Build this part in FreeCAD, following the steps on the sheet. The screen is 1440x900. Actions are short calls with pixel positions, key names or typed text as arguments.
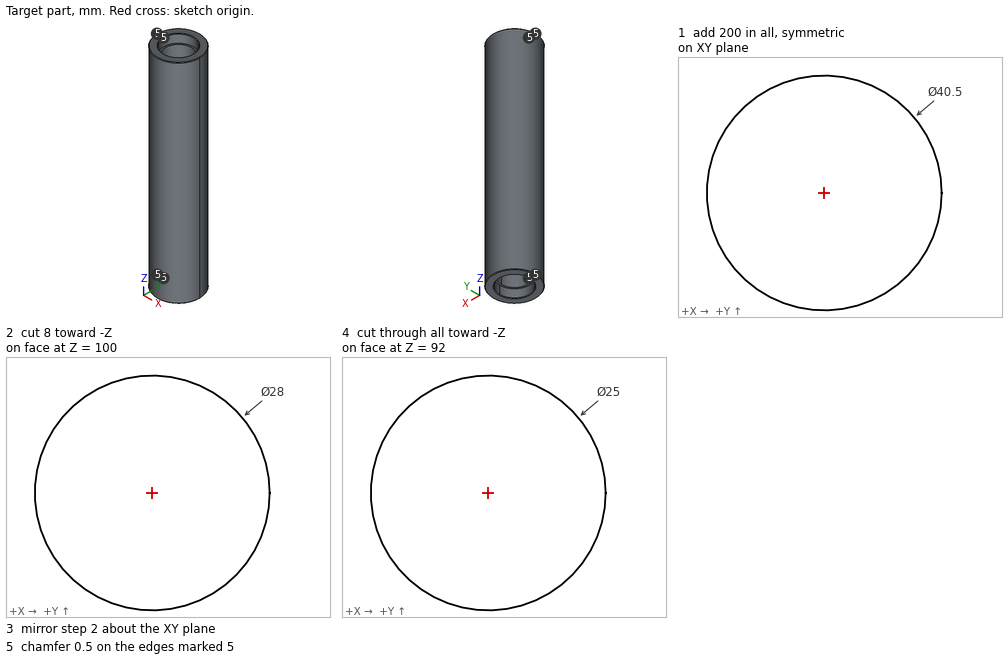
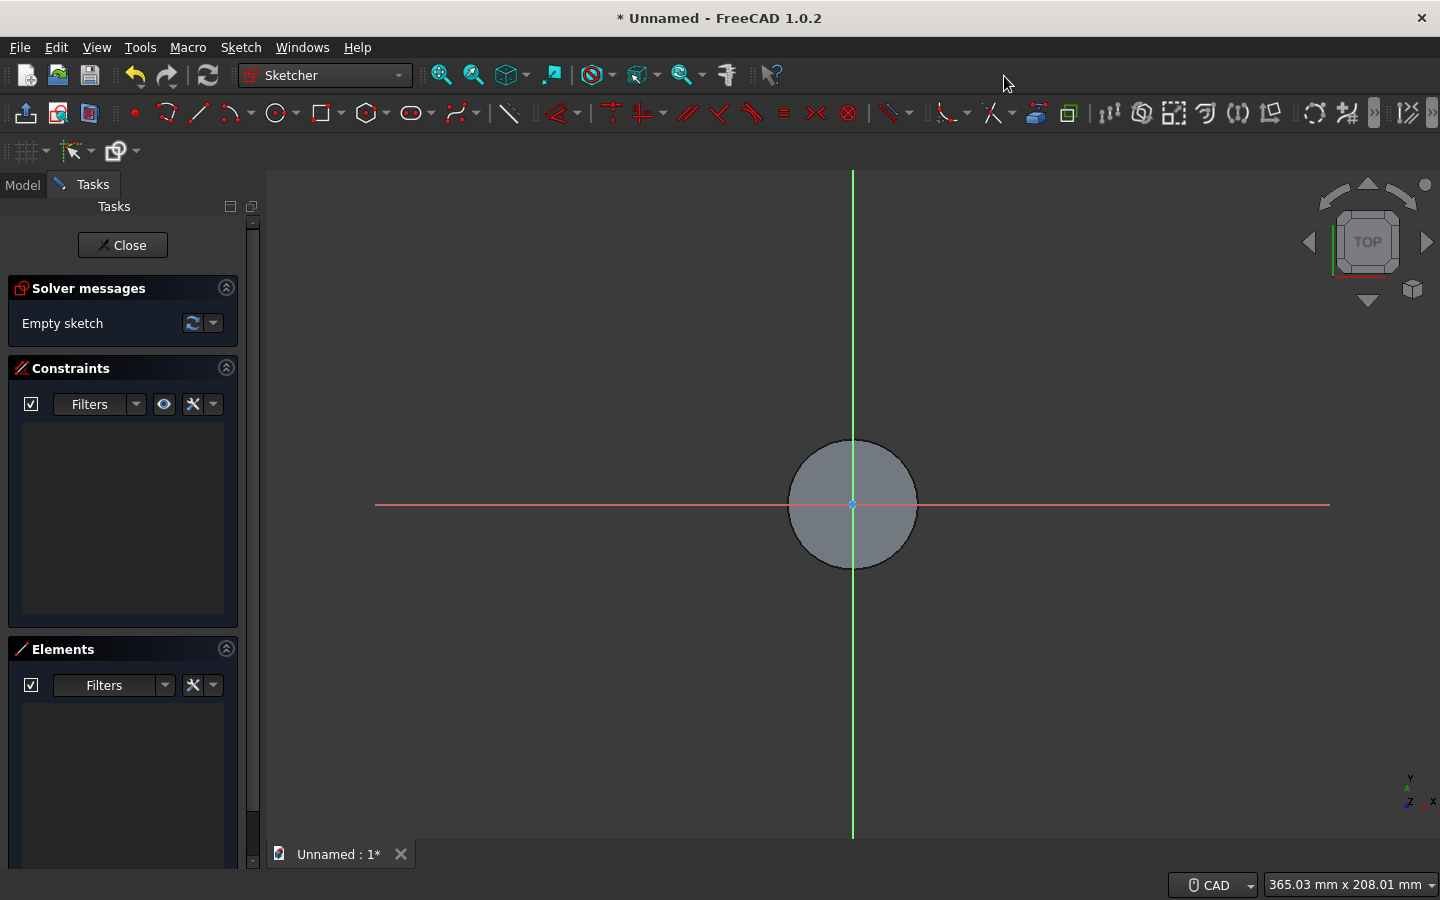
scroll(870, 504, up, 8)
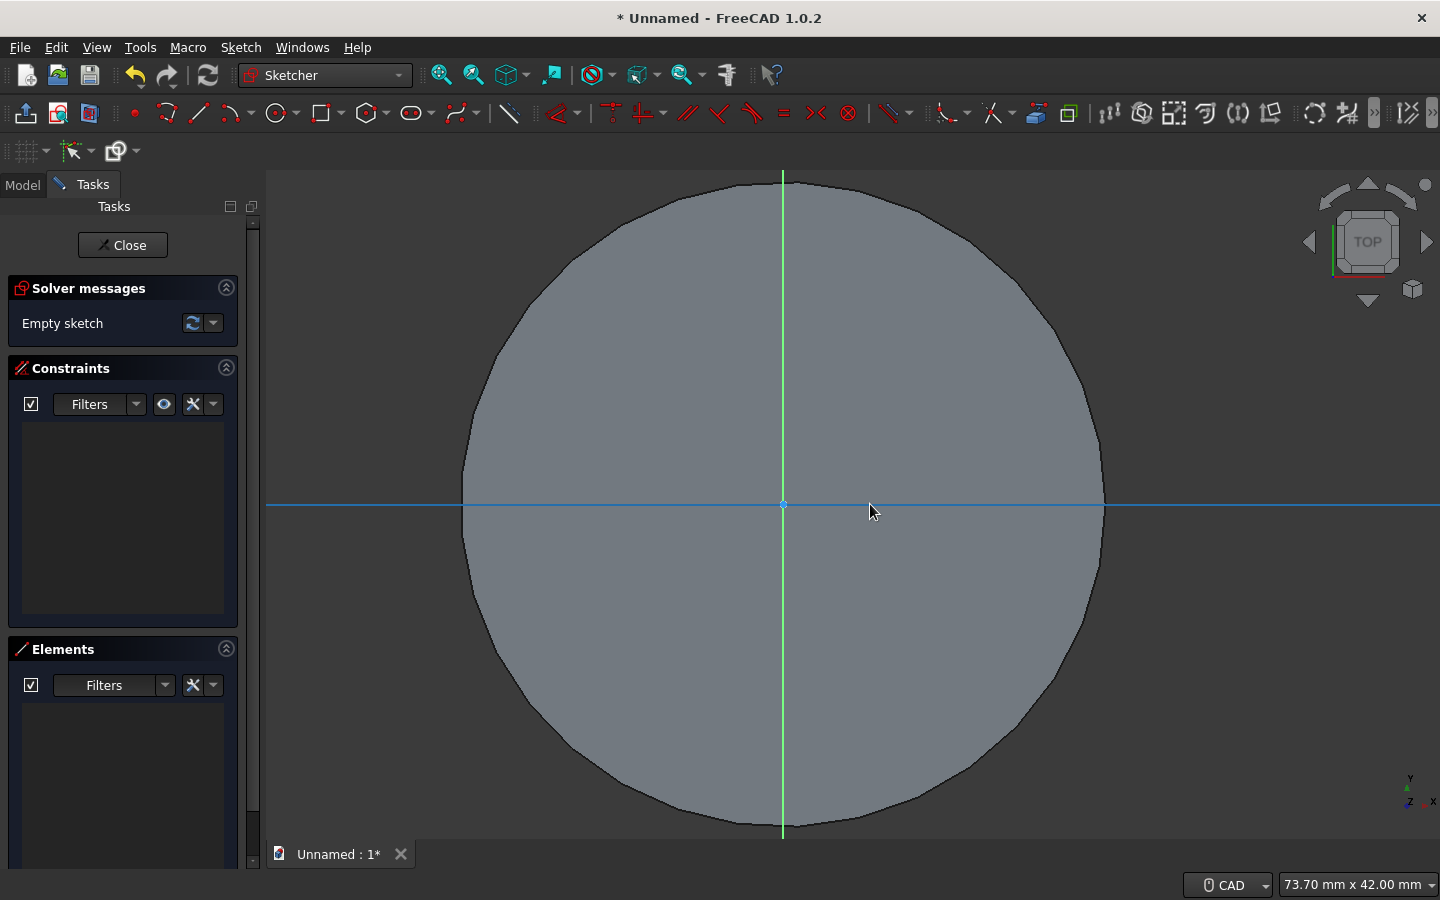
click(276, 114)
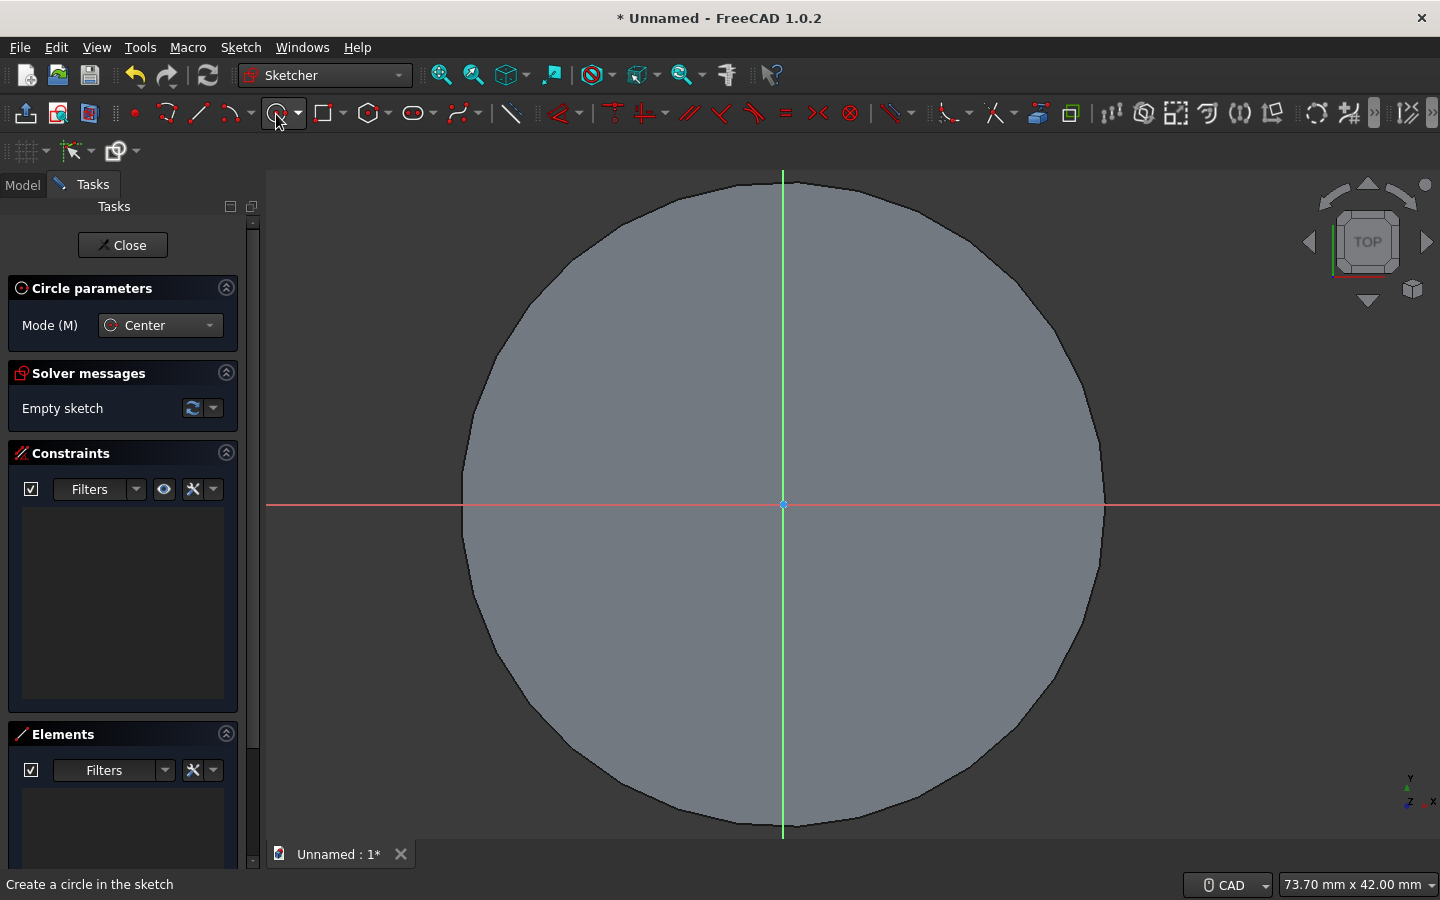
click(783, 504)
move(941, 347)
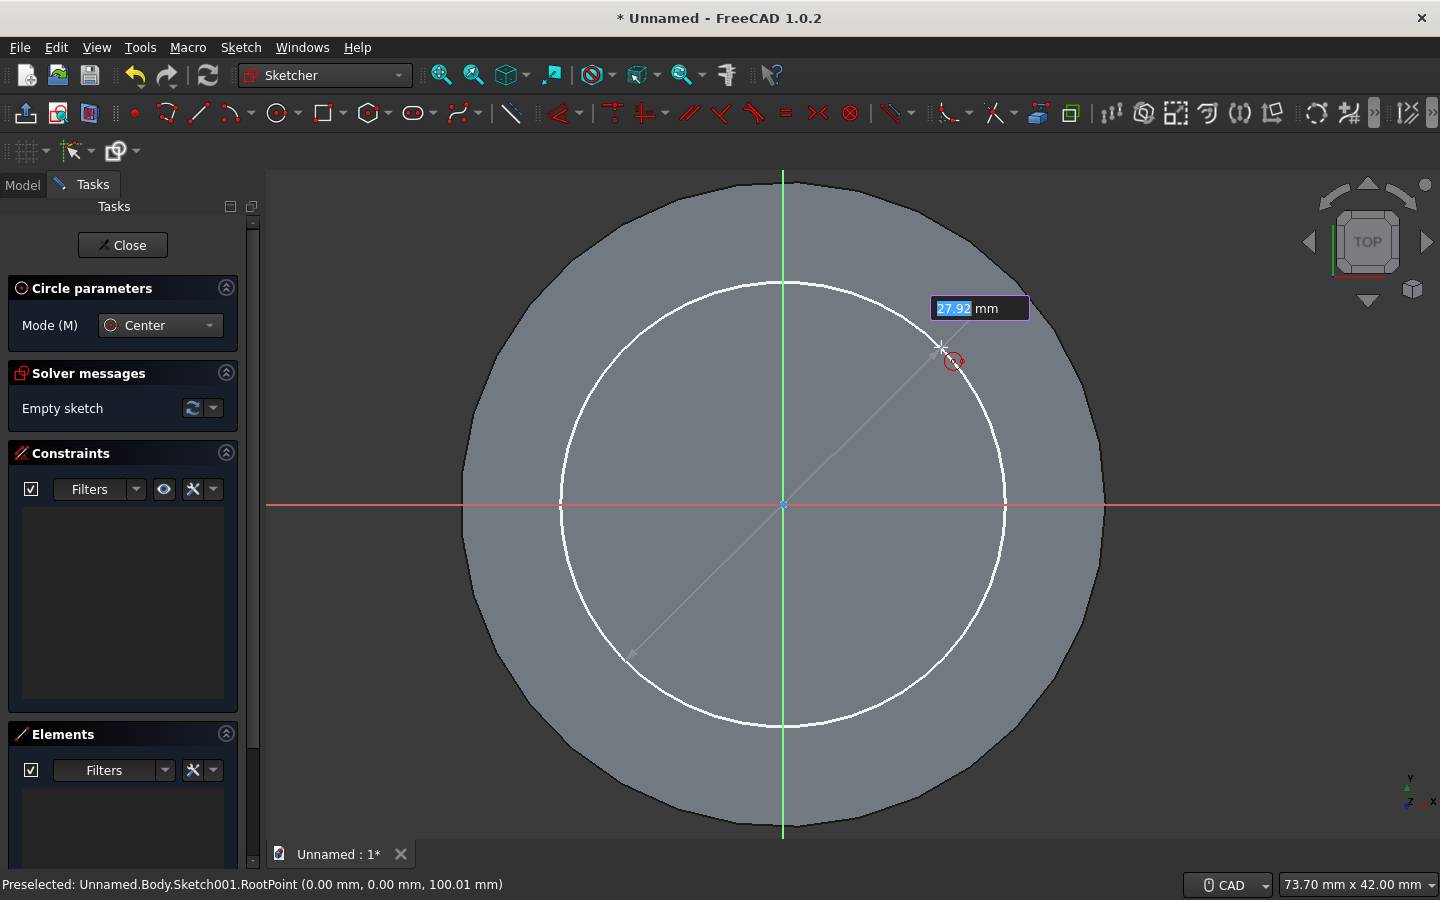
text(28)
key(Return)
key(Escape)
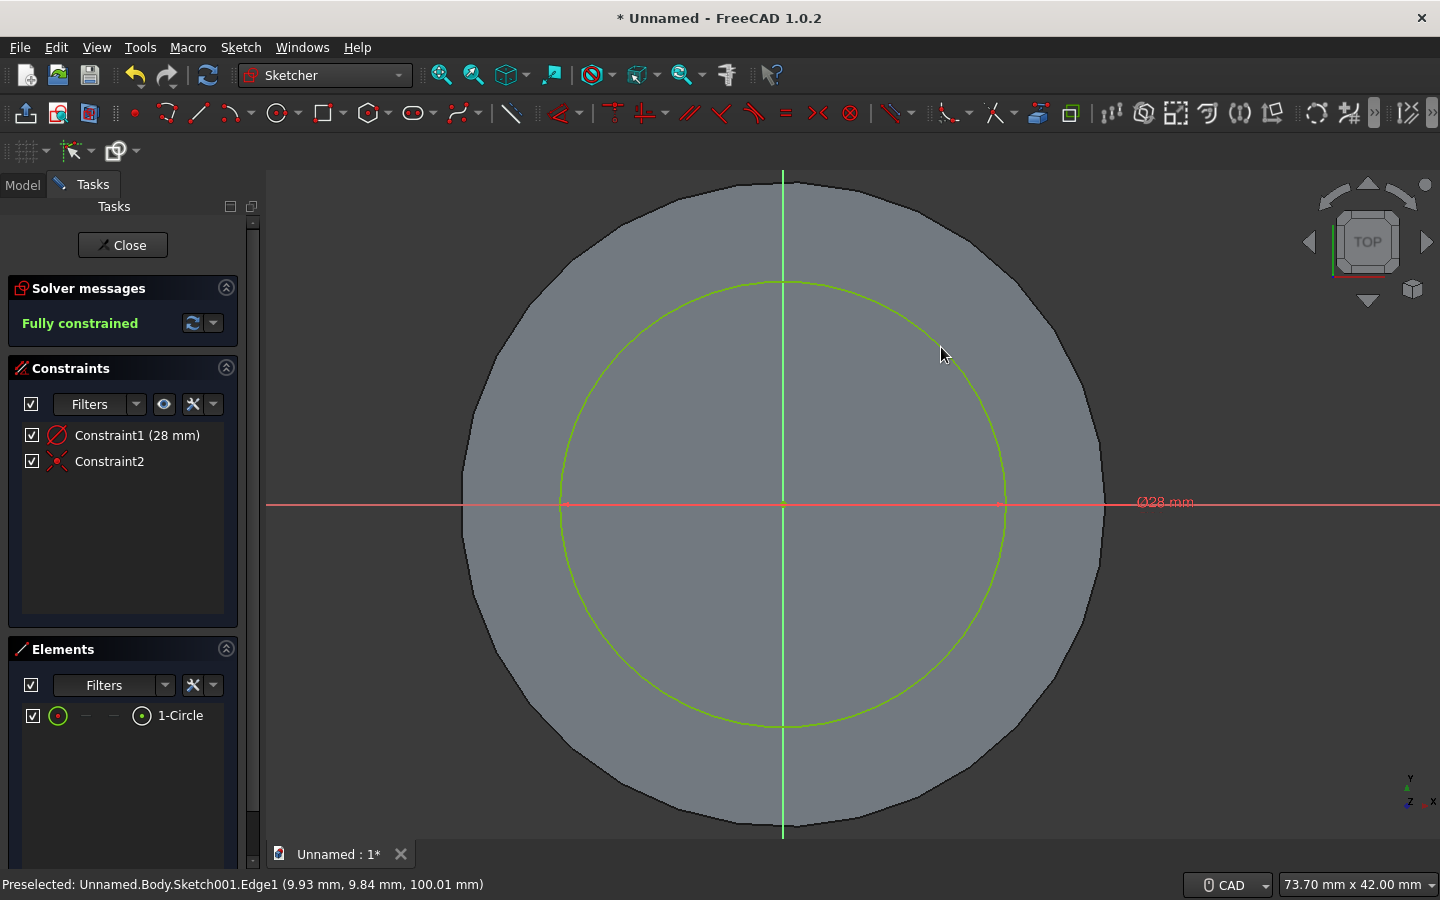
click(123, 245)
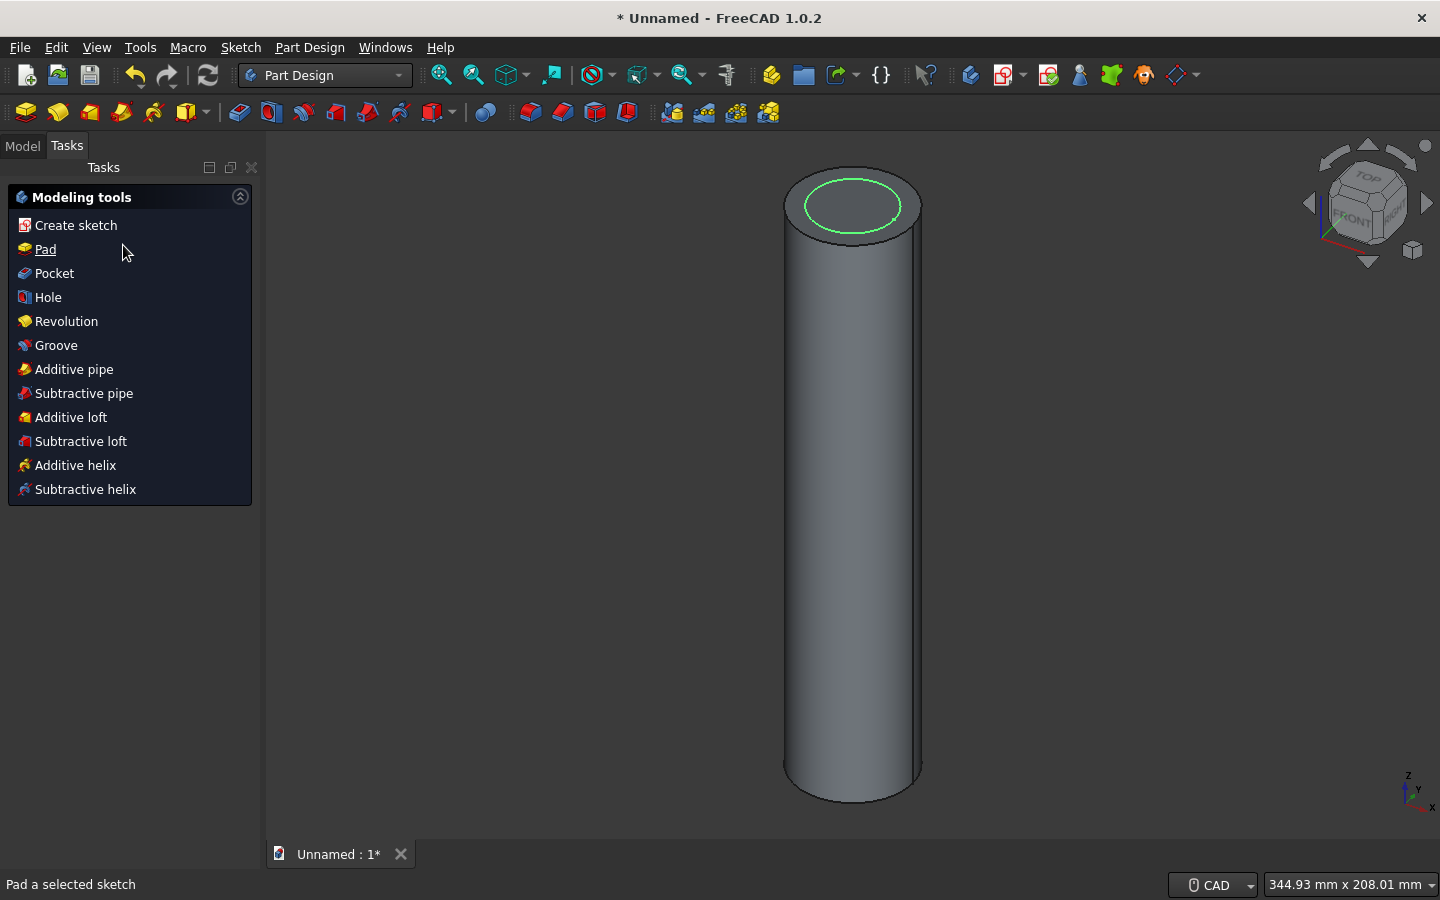
click(240, 112)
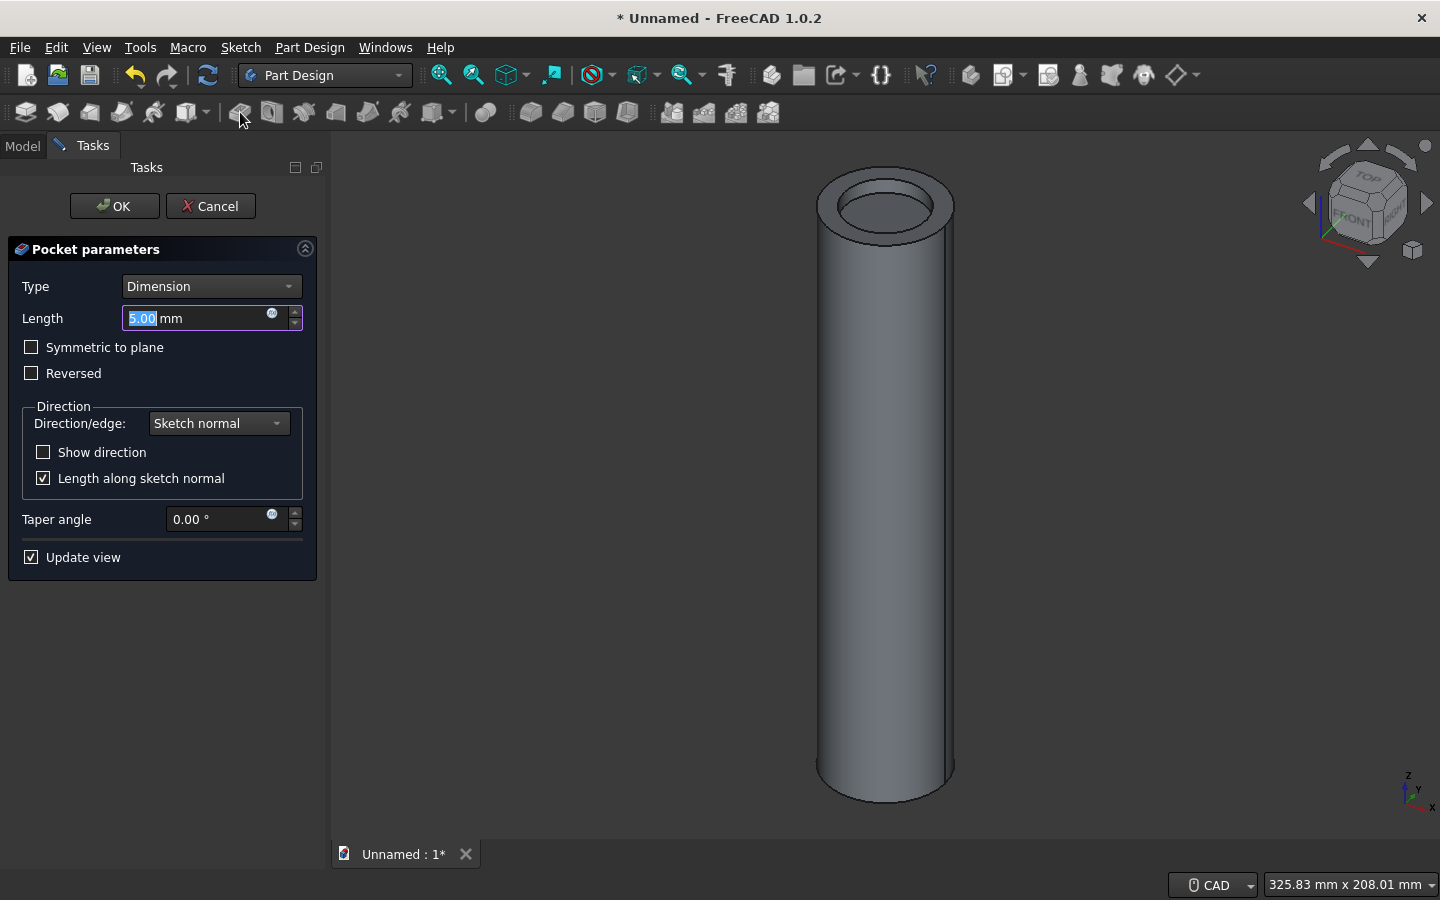
text(8)
key(Tab)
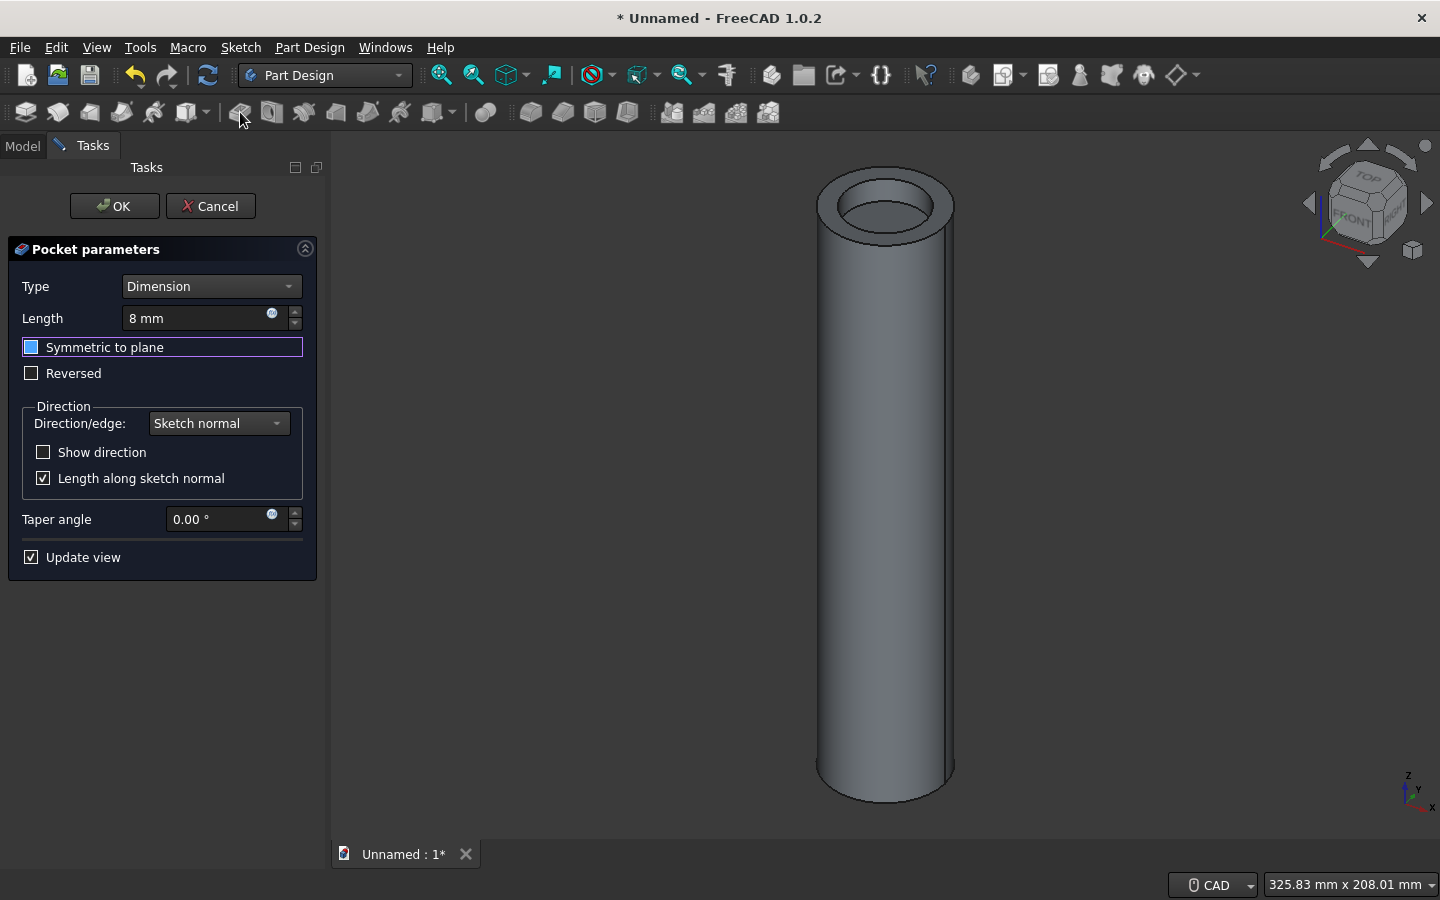
click(115, 206)